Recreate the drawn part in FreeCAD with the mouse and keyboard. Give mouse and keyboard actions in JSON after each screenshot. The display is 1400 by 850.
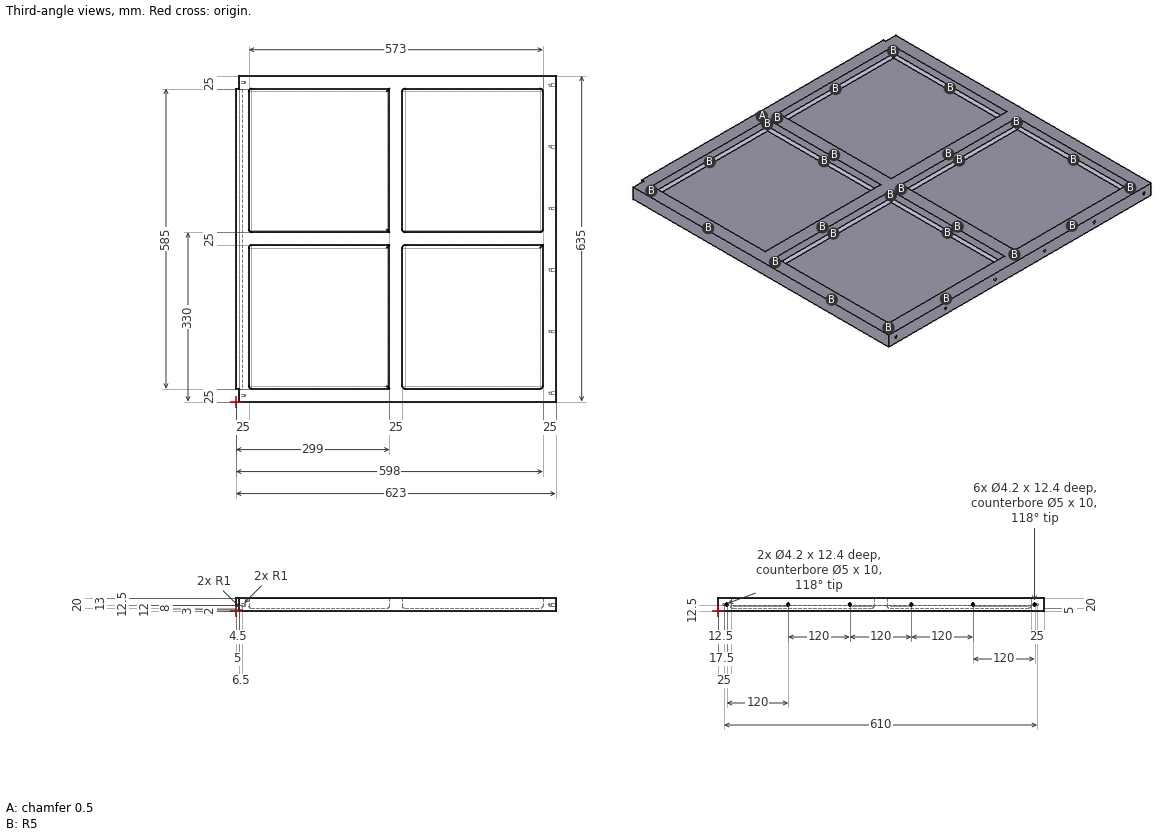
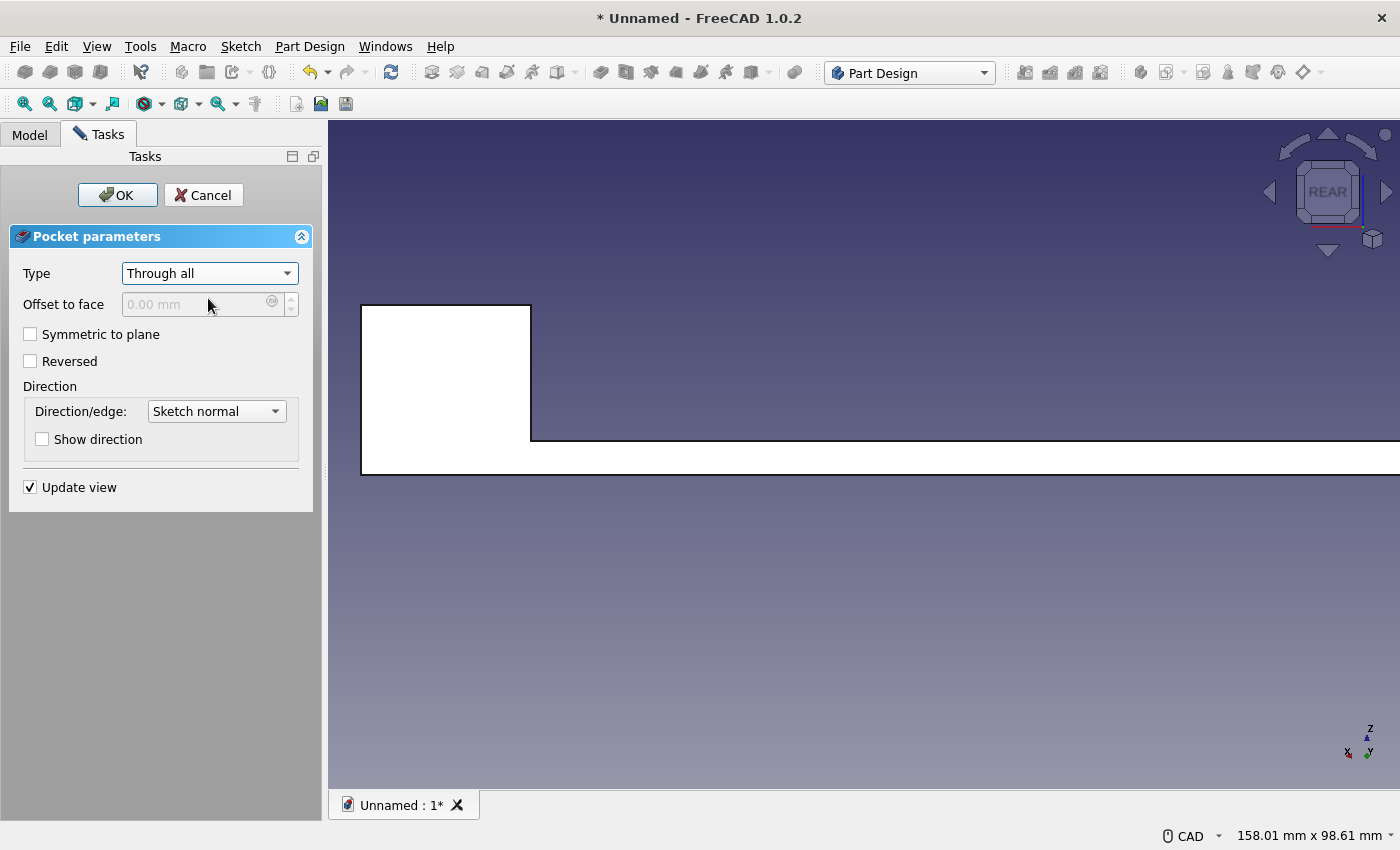
{"action": "left_click", "coordinate": [118, 195]}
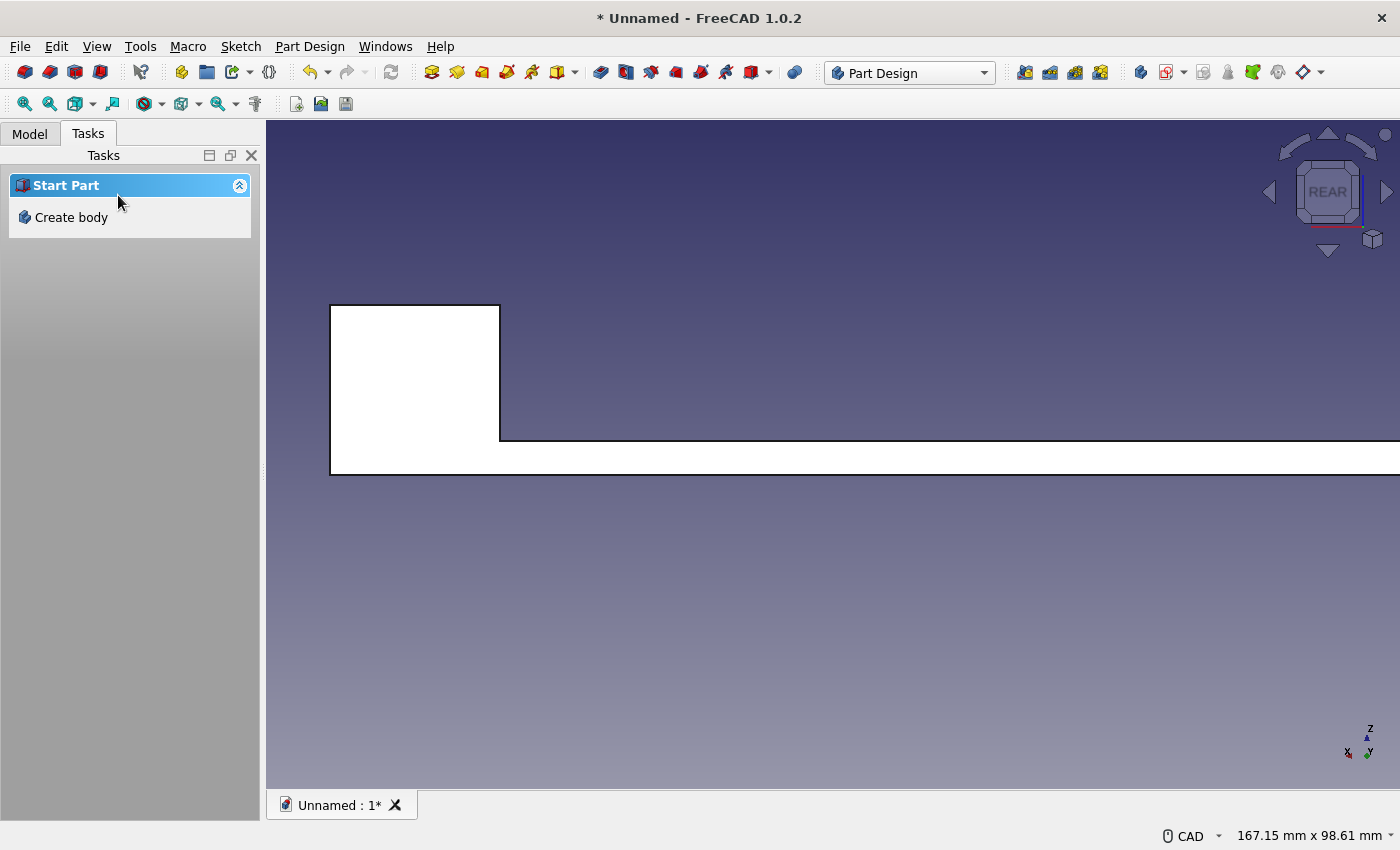
{"action": "left_click", "coordinate": [25, 104]}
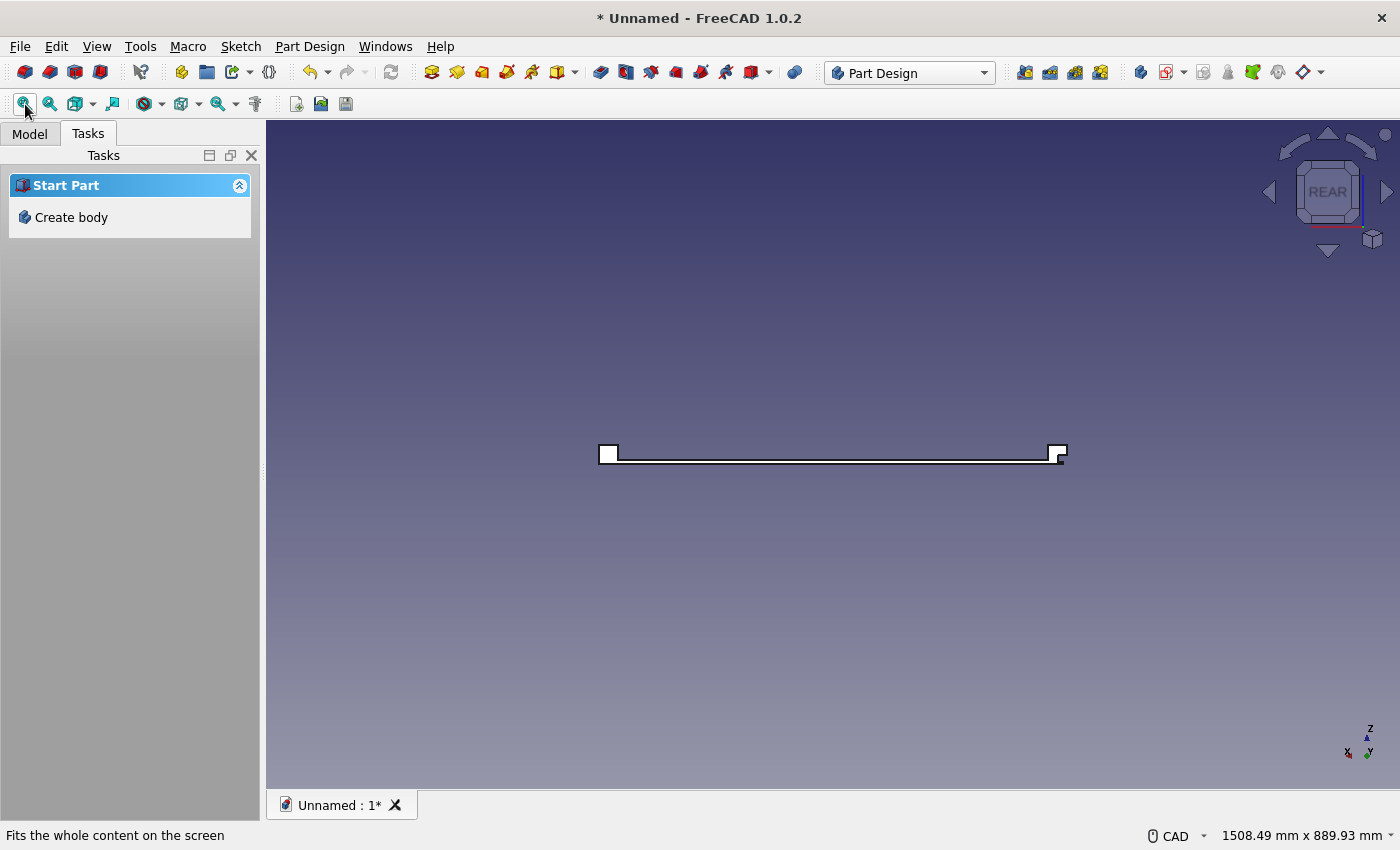
{"action": "key", "text": "0"}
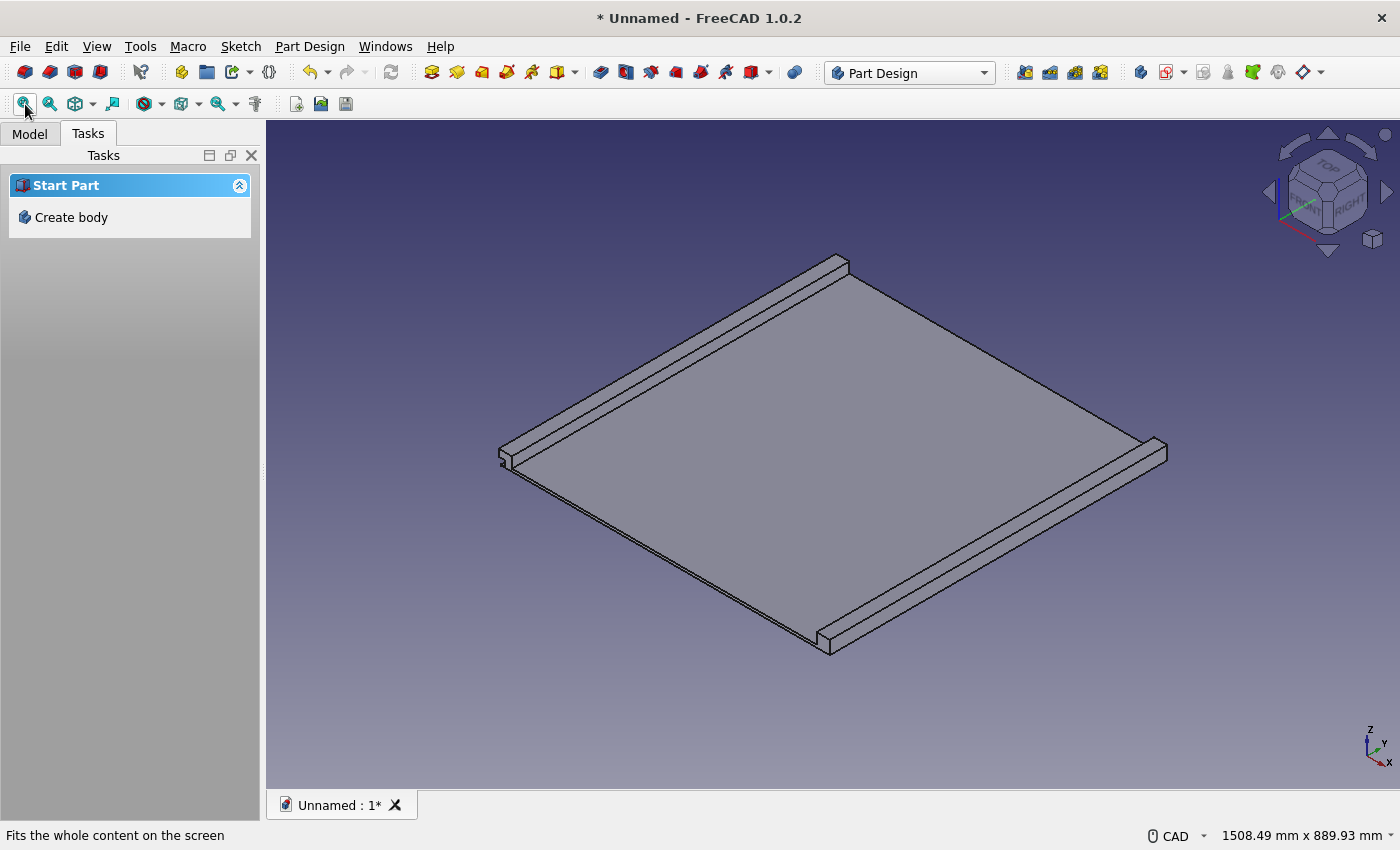
{"action": "key", "text": "2"}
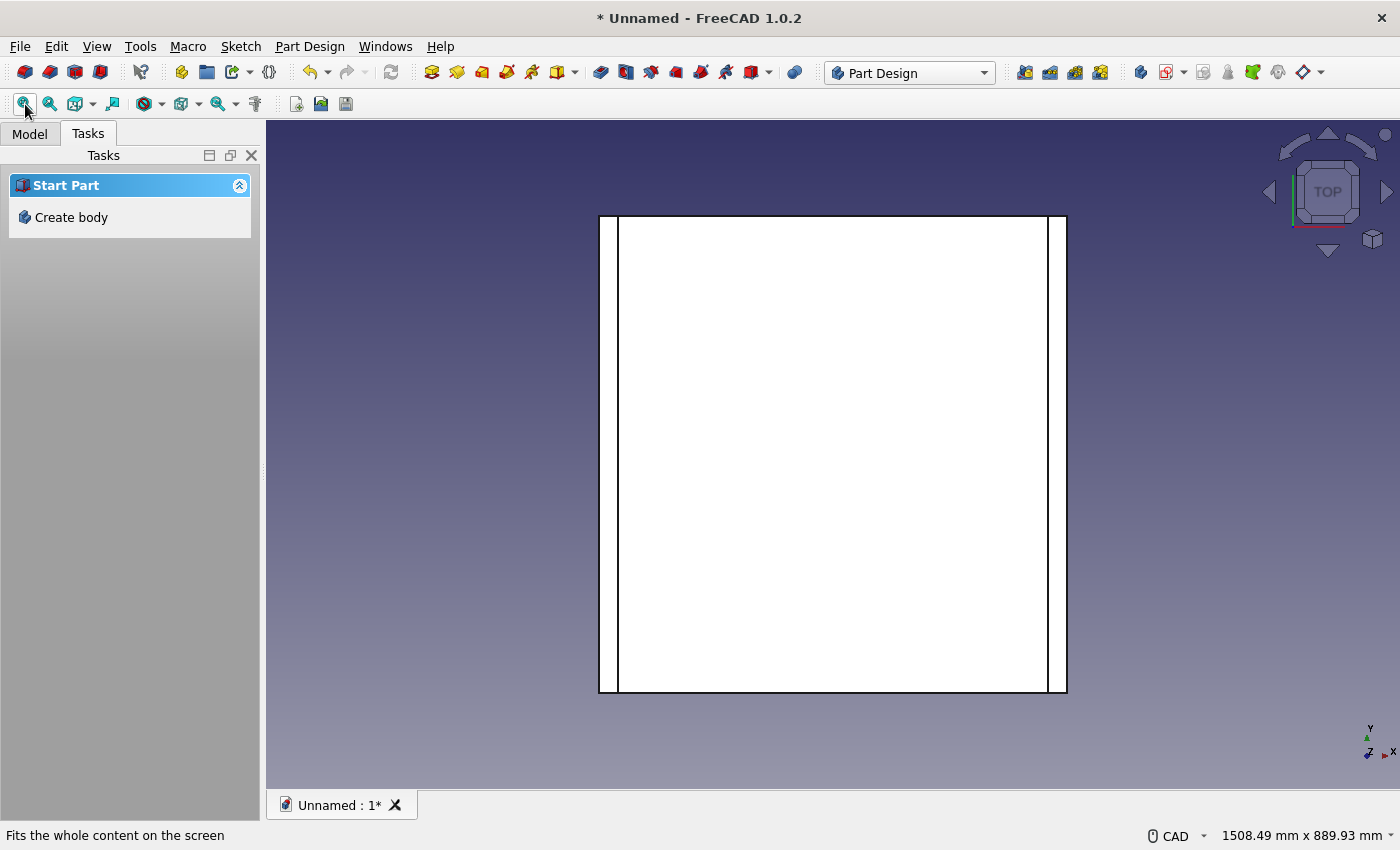
{"action": "key", "text": "1"}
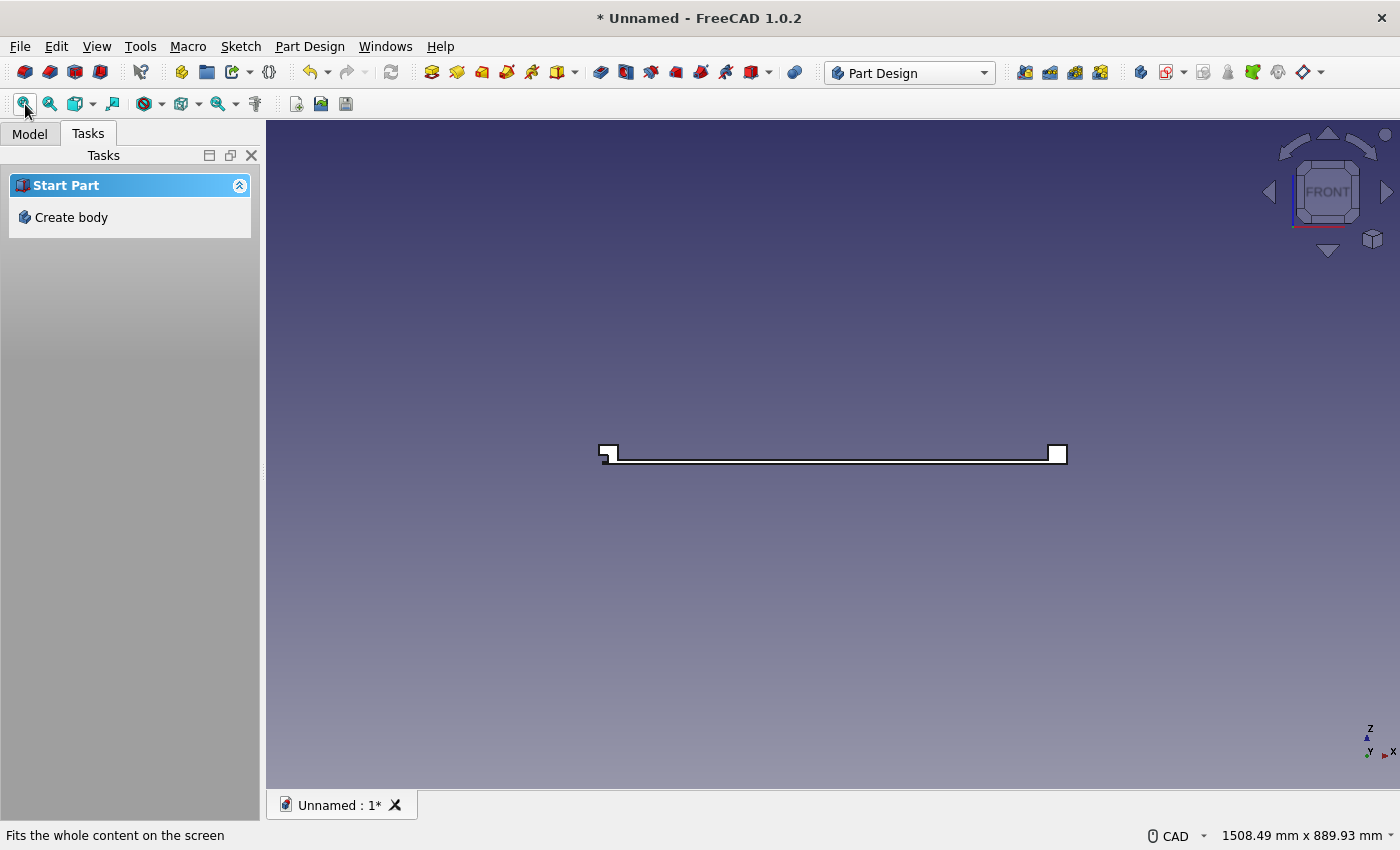
{"action": "left_click", "coordinate": [25, 104]}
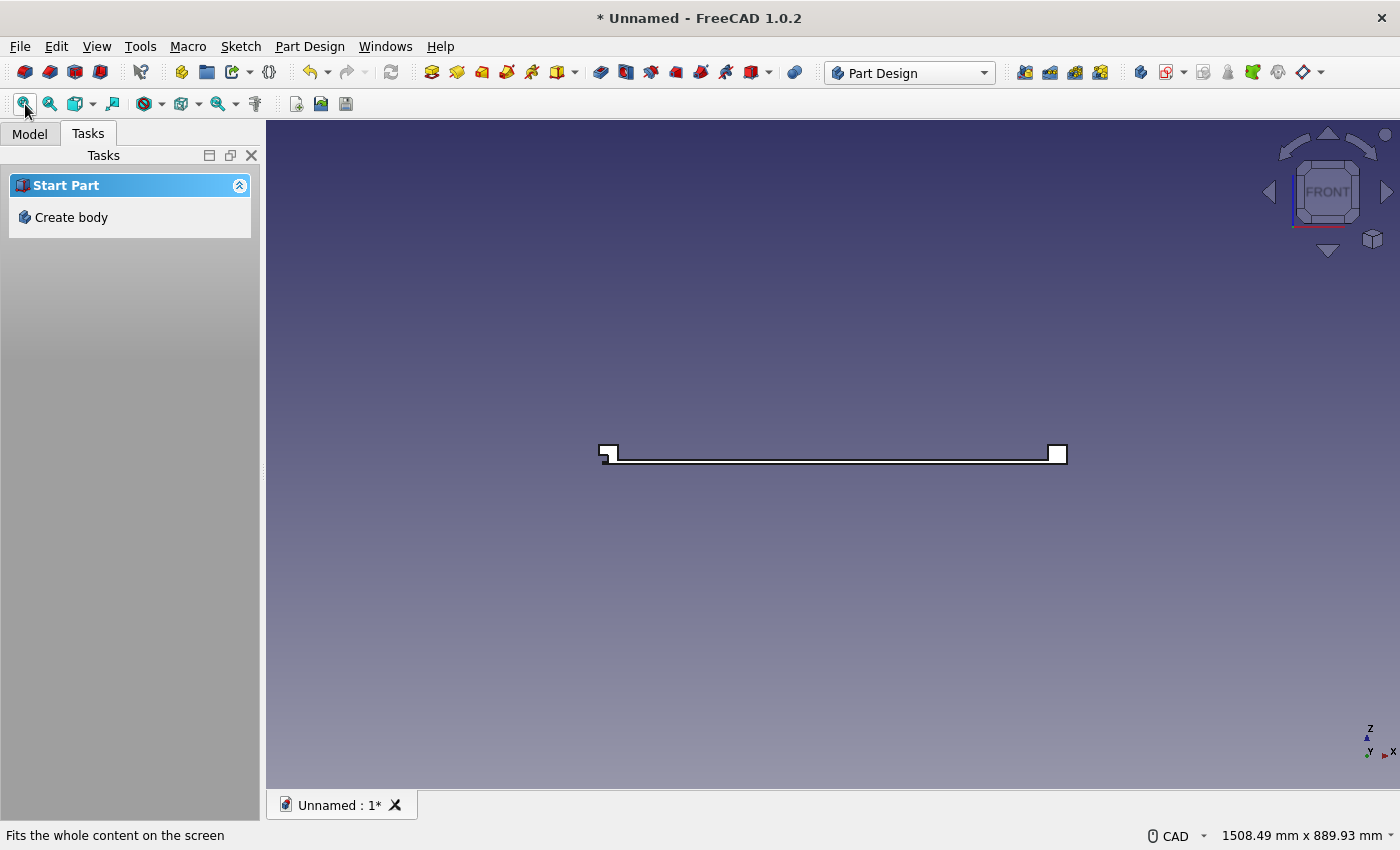
{"action": "key", "text": "3"}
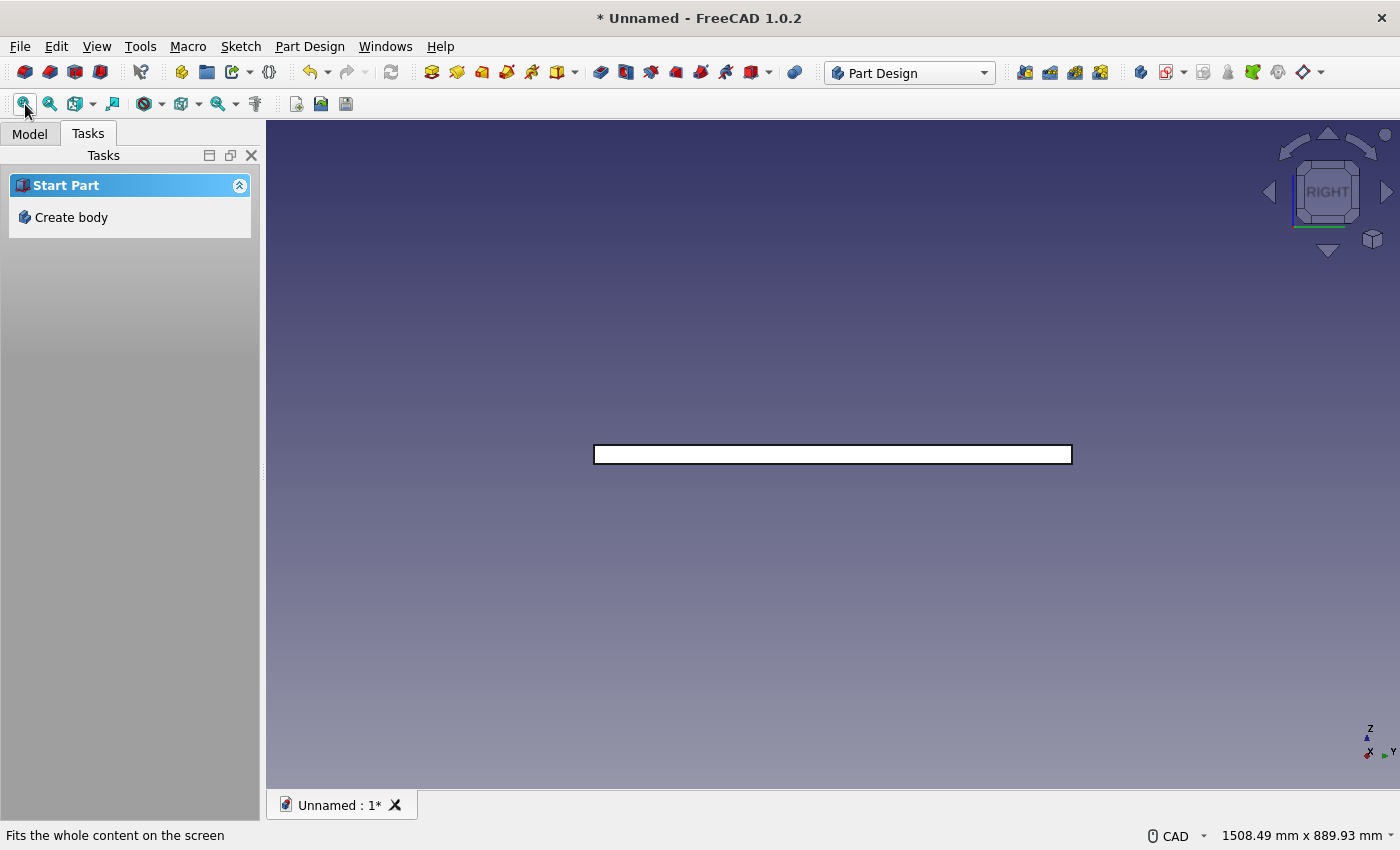
{"action": "left_click", "coordinate": [25, 104]}